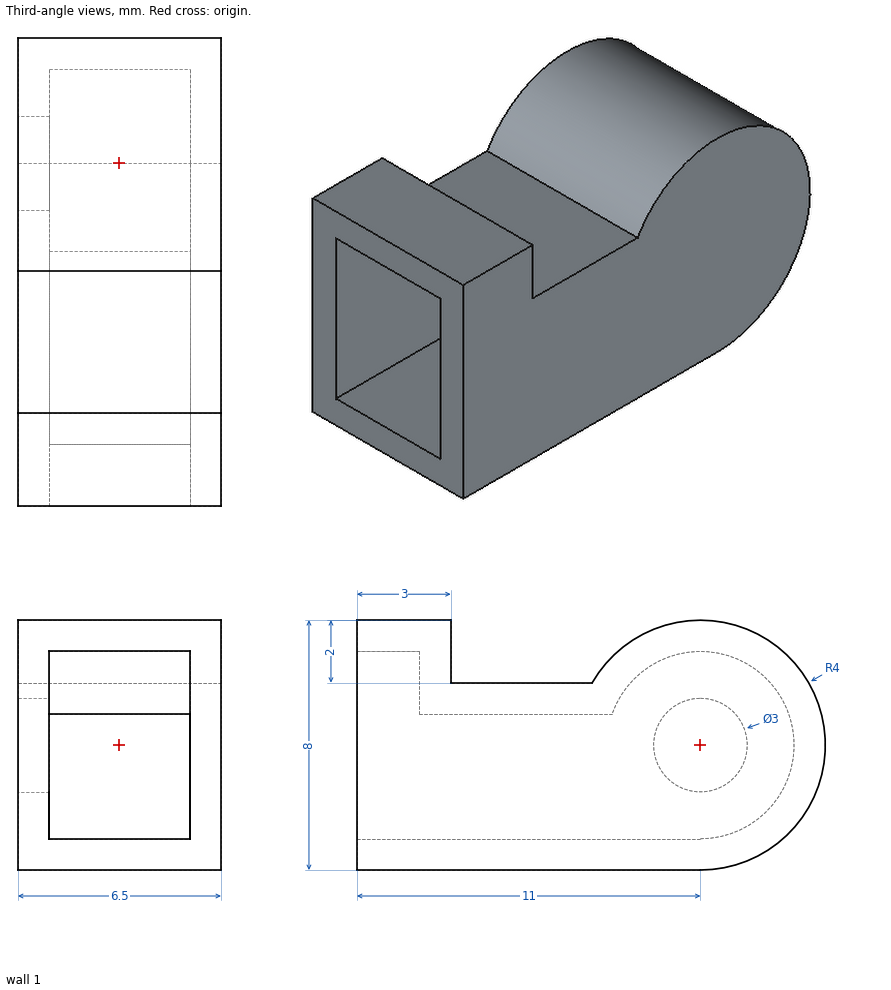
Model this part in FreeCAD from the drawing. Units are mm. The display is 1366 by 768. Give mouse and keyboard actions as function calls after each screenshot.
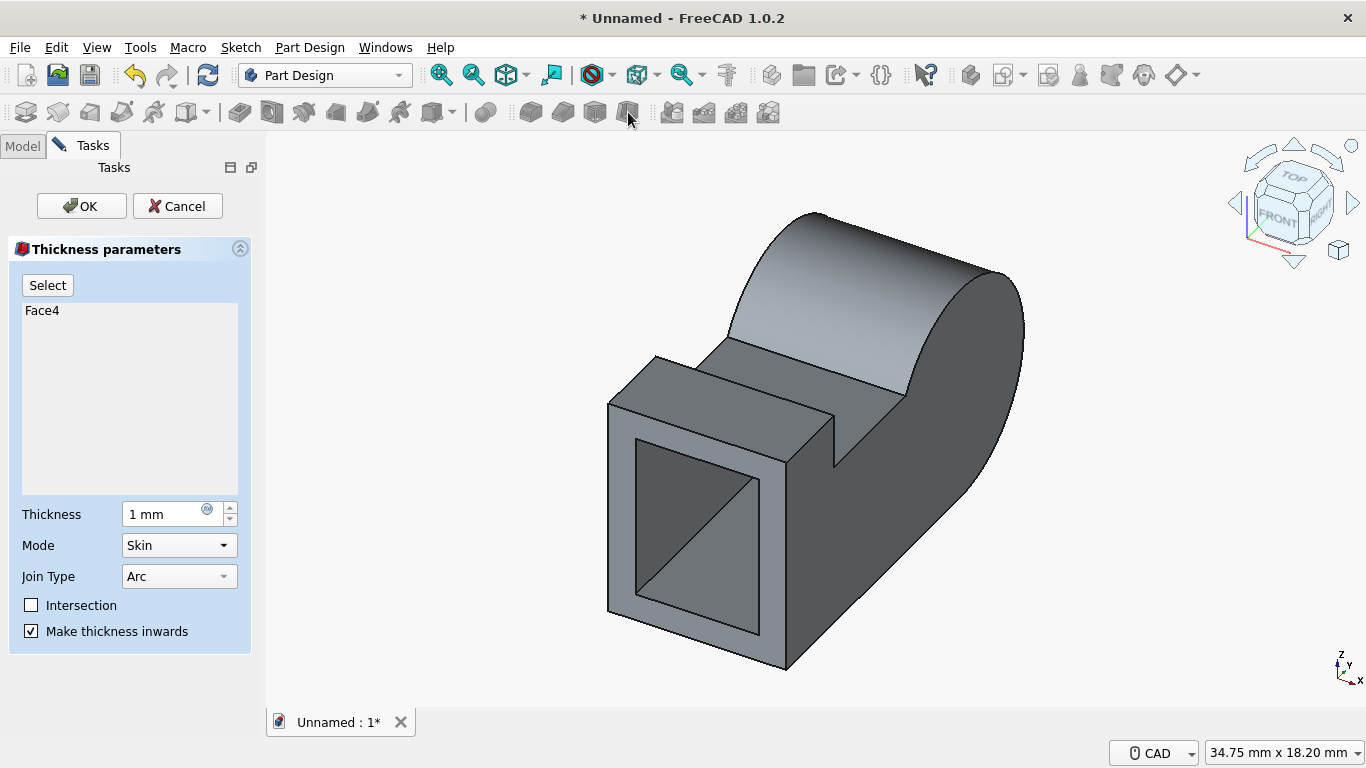
click(180, 576)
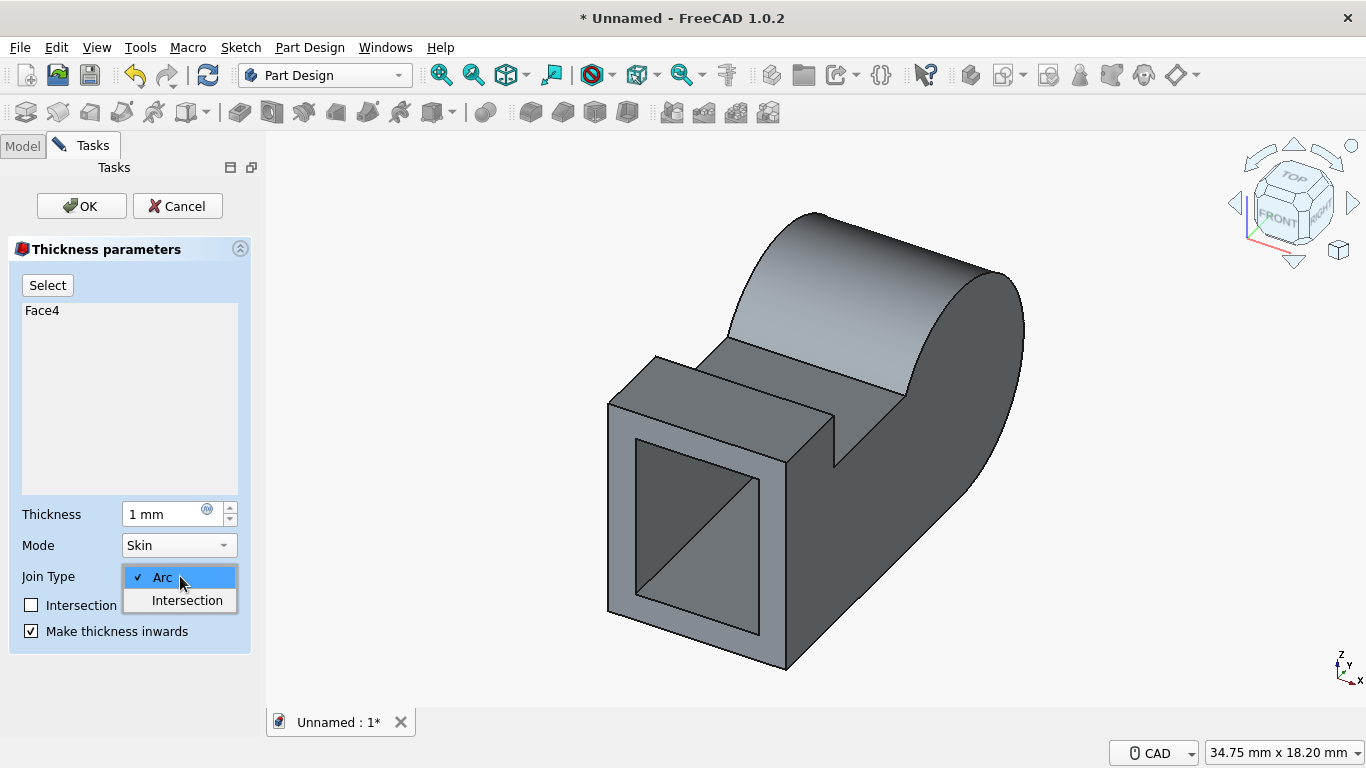
click(179, 600)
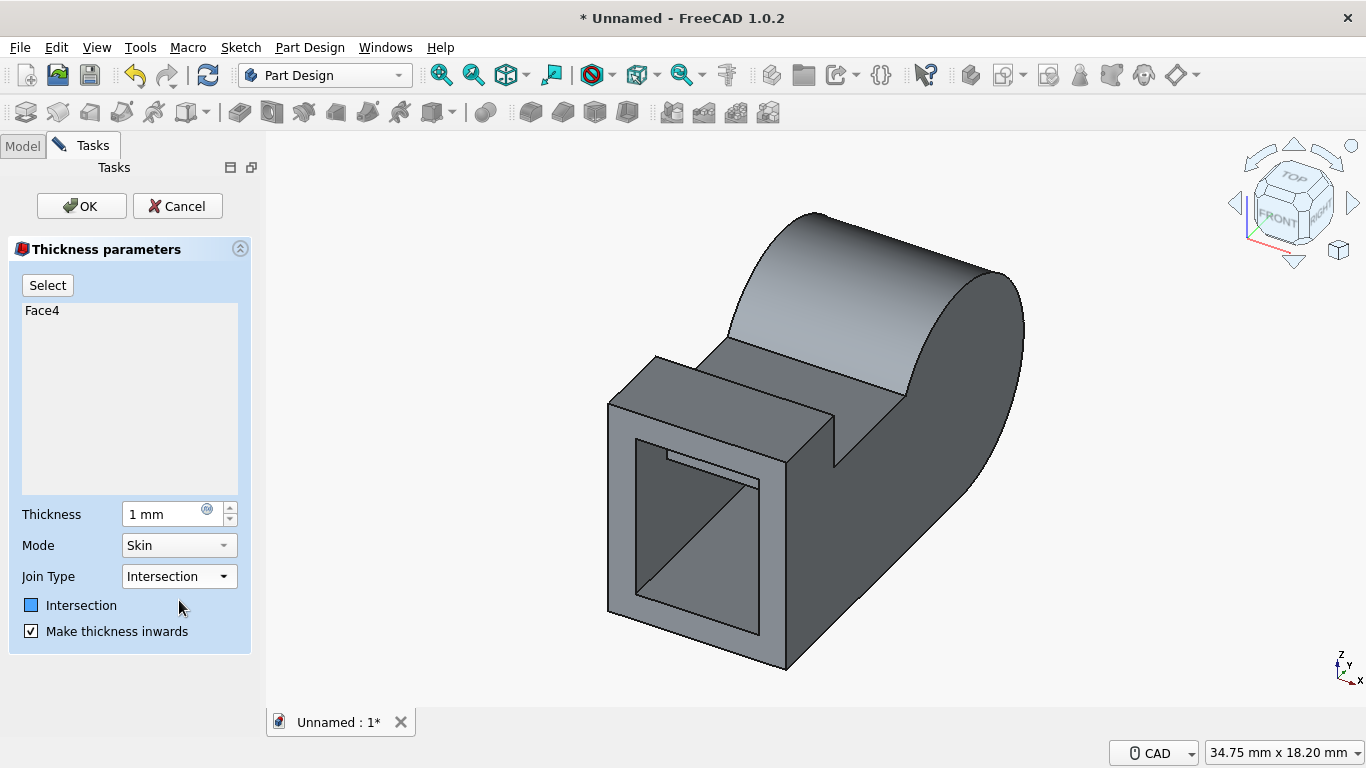
click(82, 206)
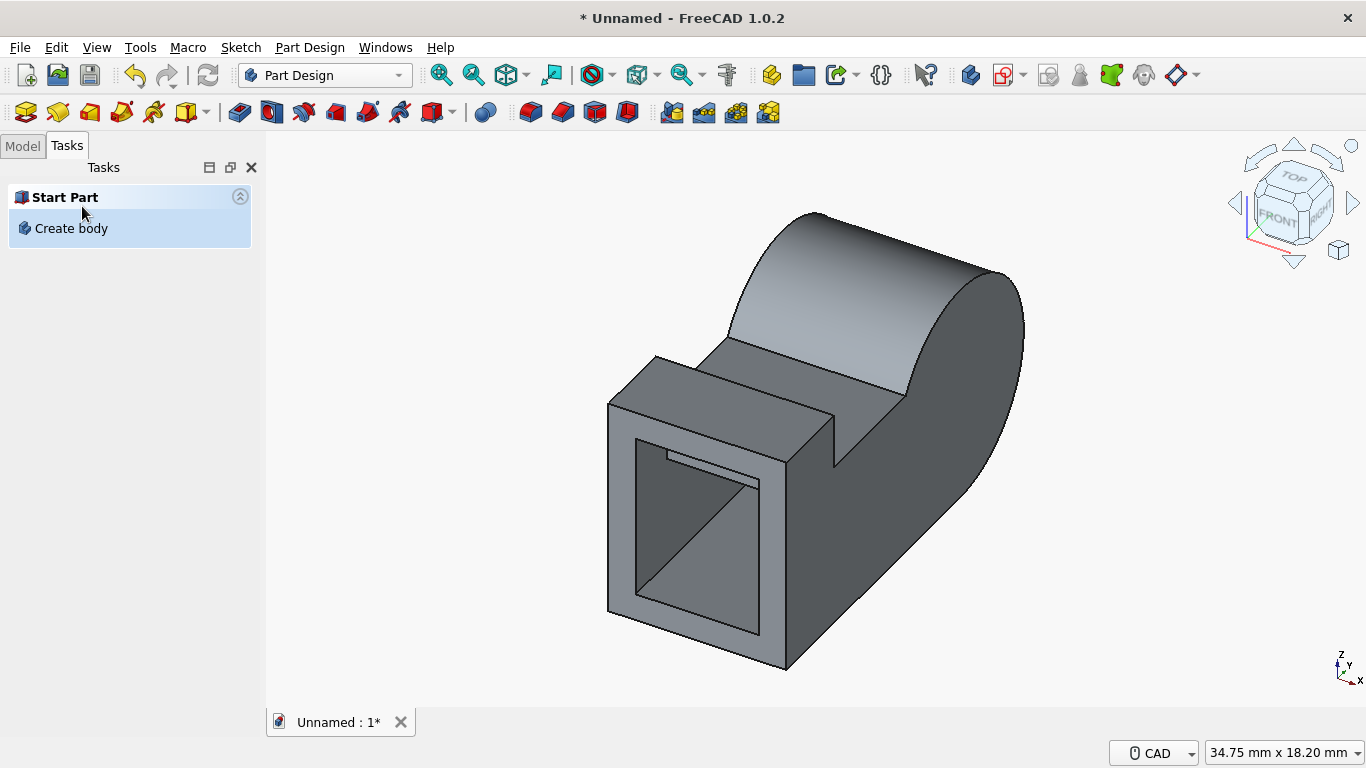
key(6)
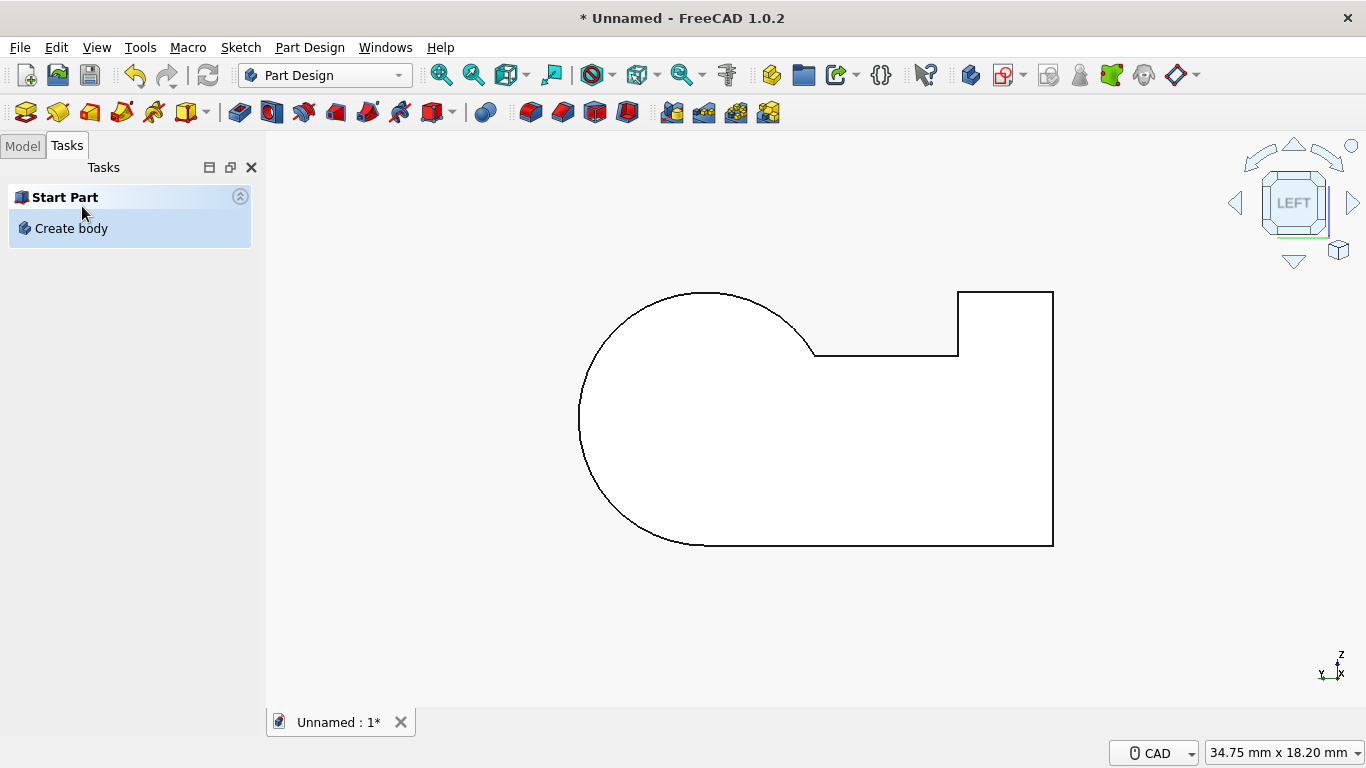
key(v)
key(f)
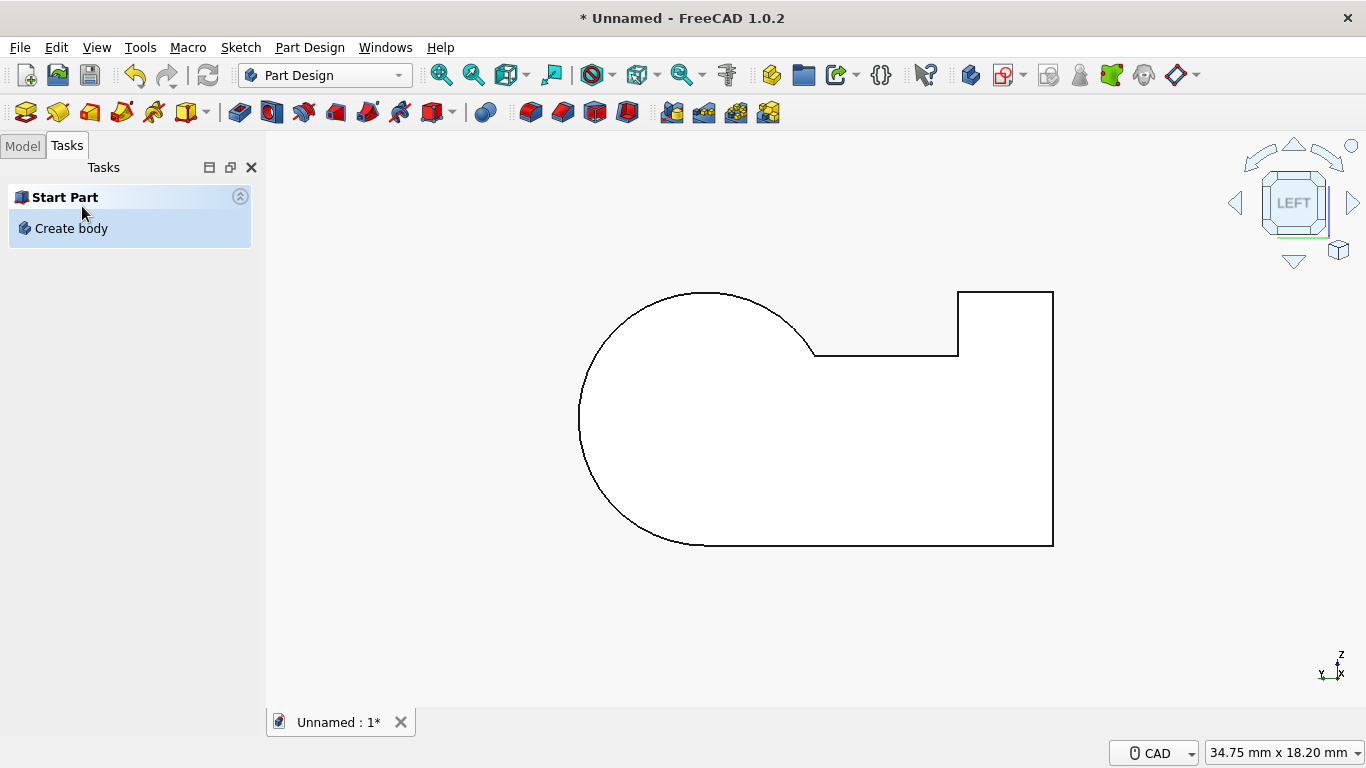
click(680, 418)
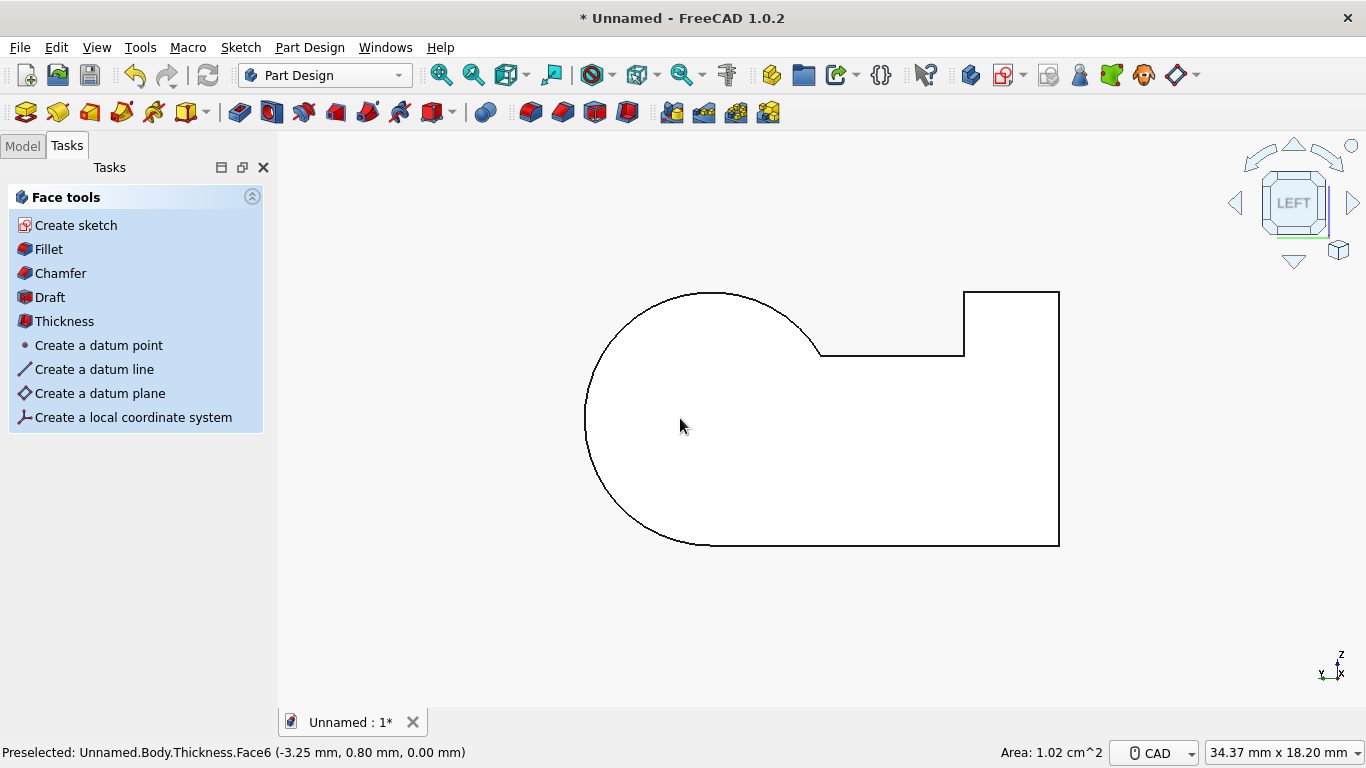
click(1004, 76)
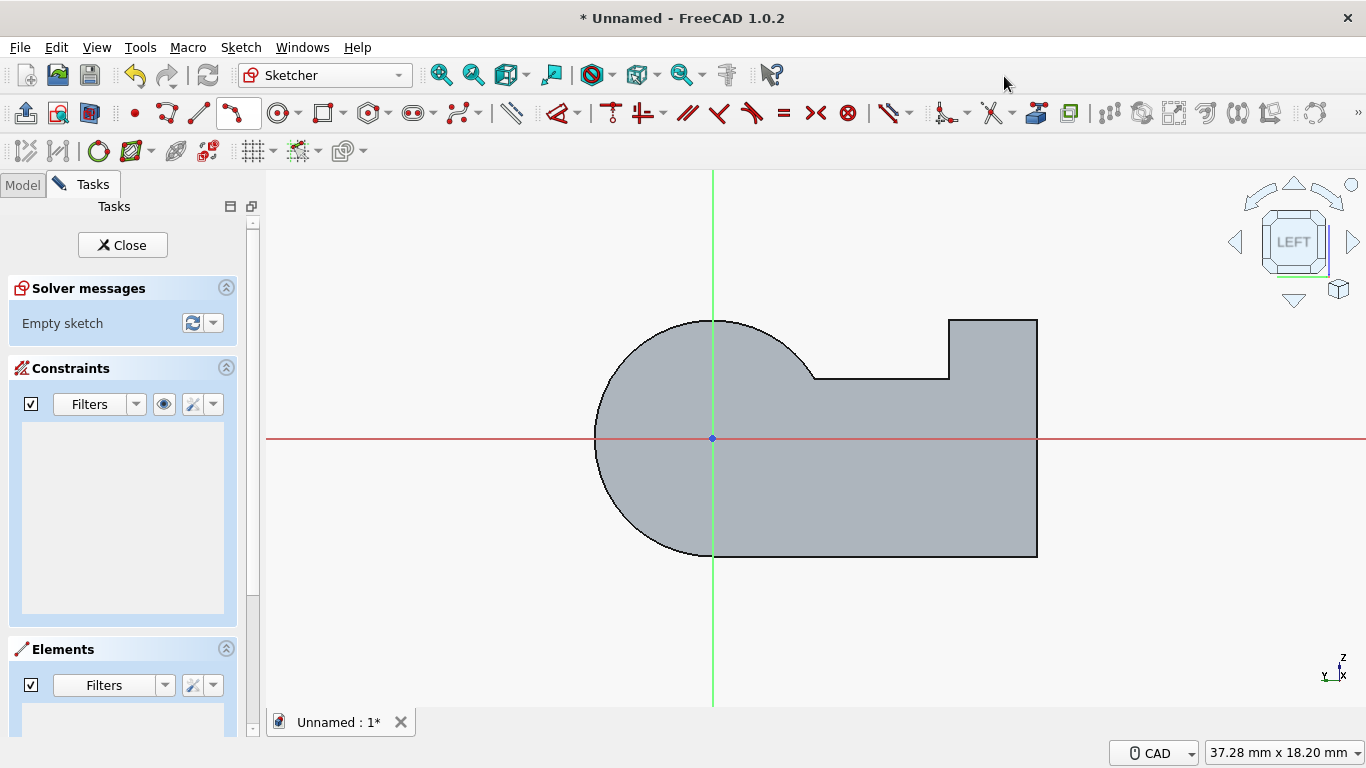
scroll(701, 438, up, 7)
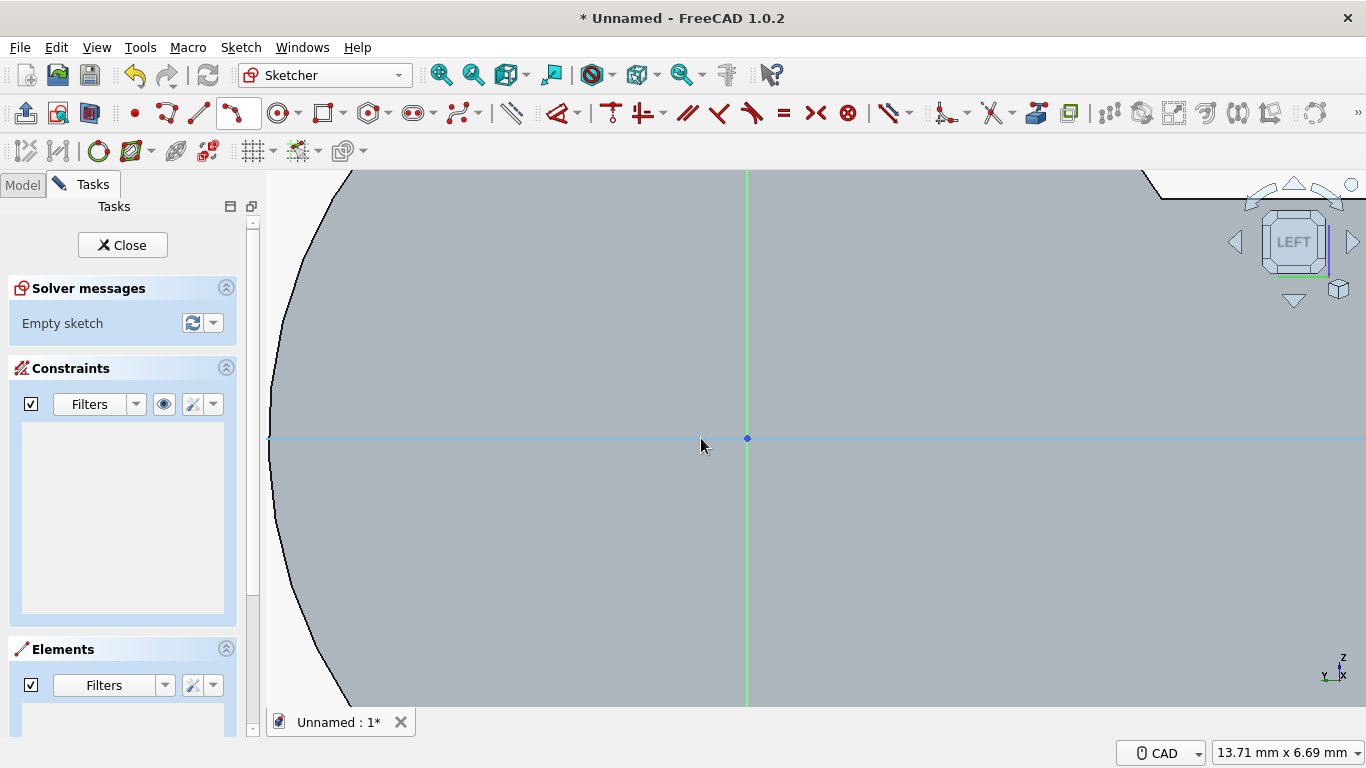
key(g)
key(c)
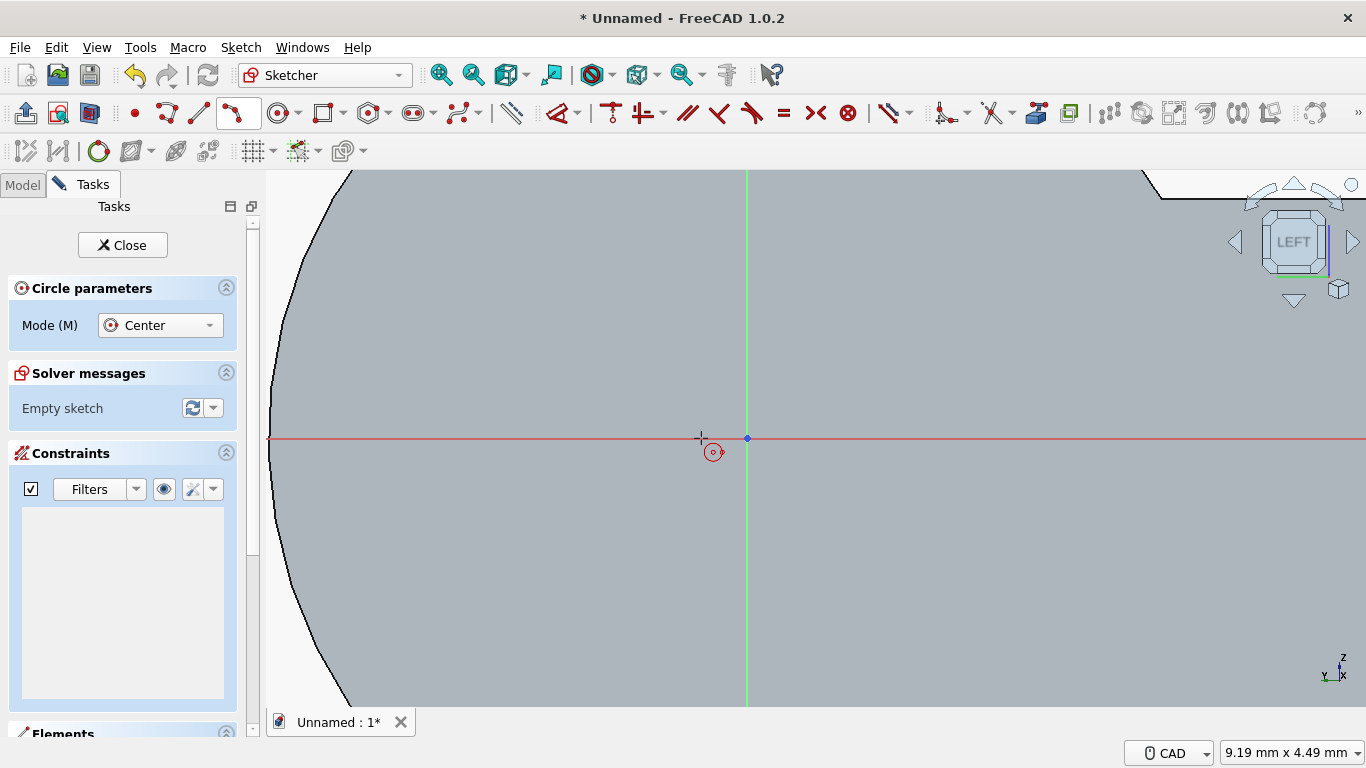
click(747, 439)
click(874, 312)
key(Escape)